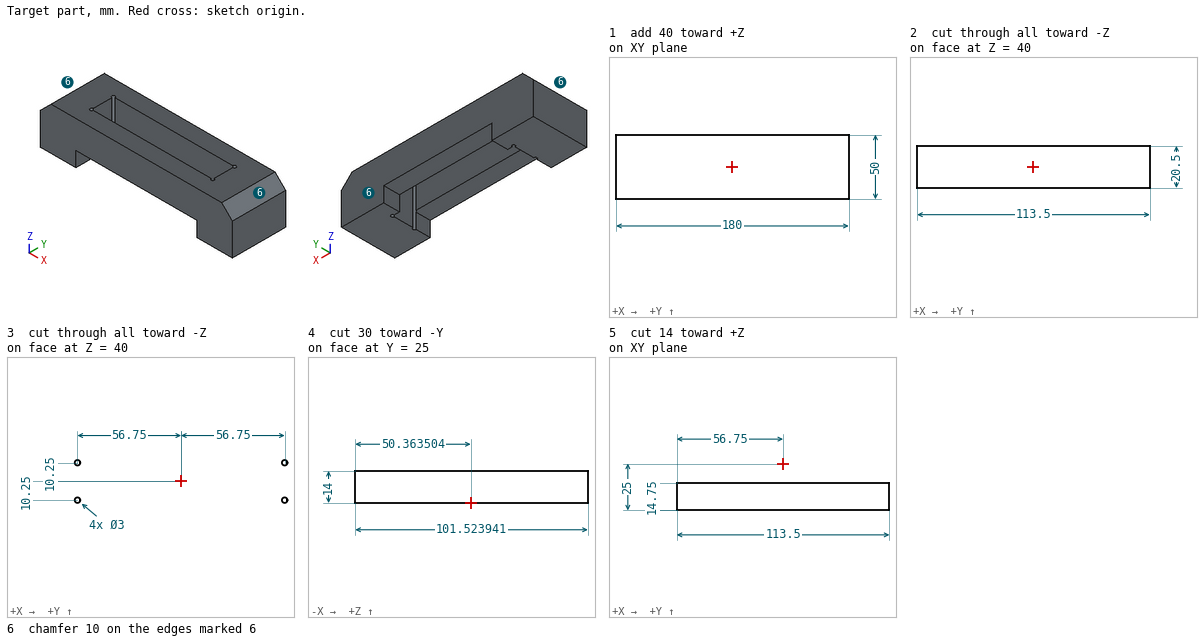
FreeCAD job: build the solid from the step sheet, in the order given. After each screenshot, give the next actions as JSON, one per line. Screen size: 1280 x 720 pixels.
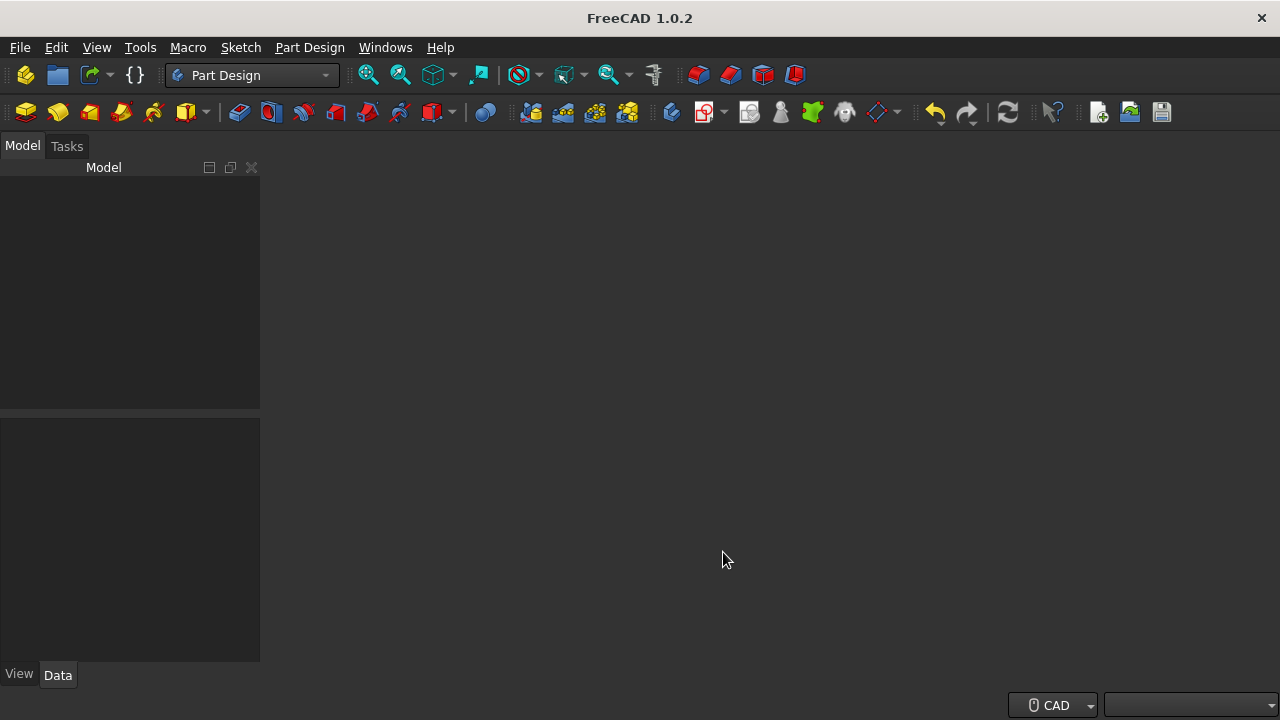
{"action": "left_click", "coordinate": [1098, 112]}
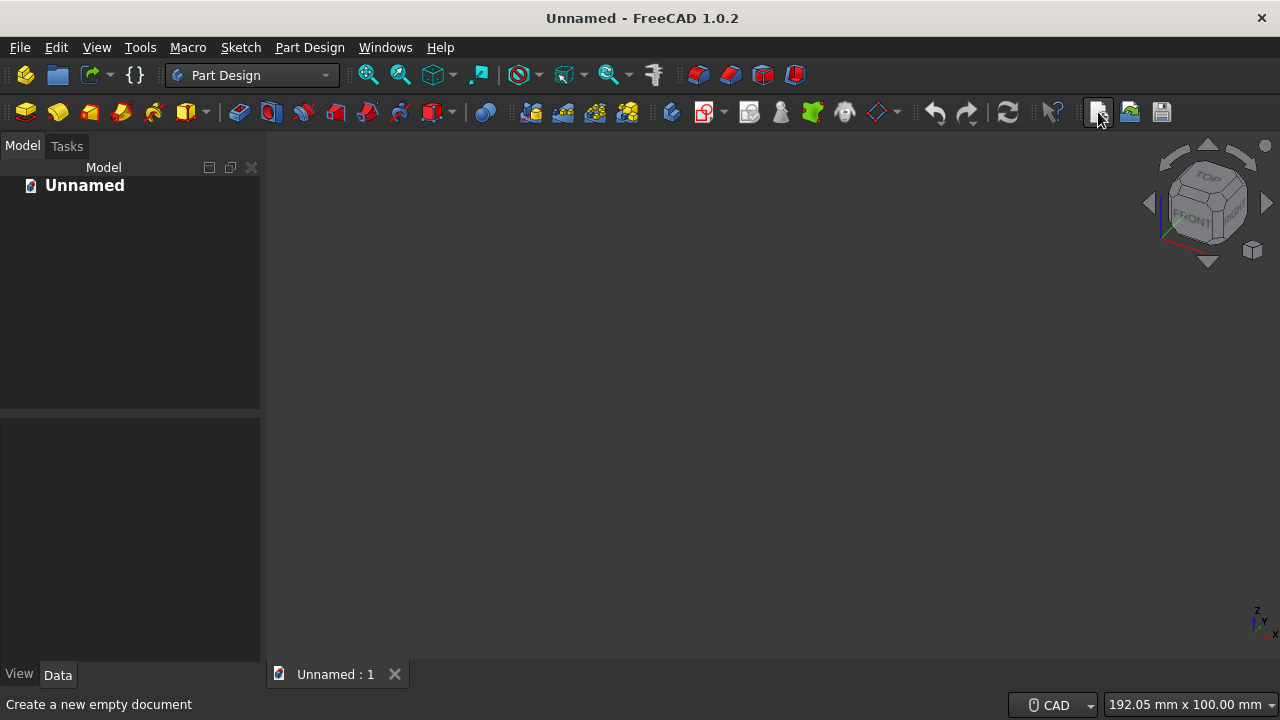
{"action": "left_click", "coordinate": [704, 112]}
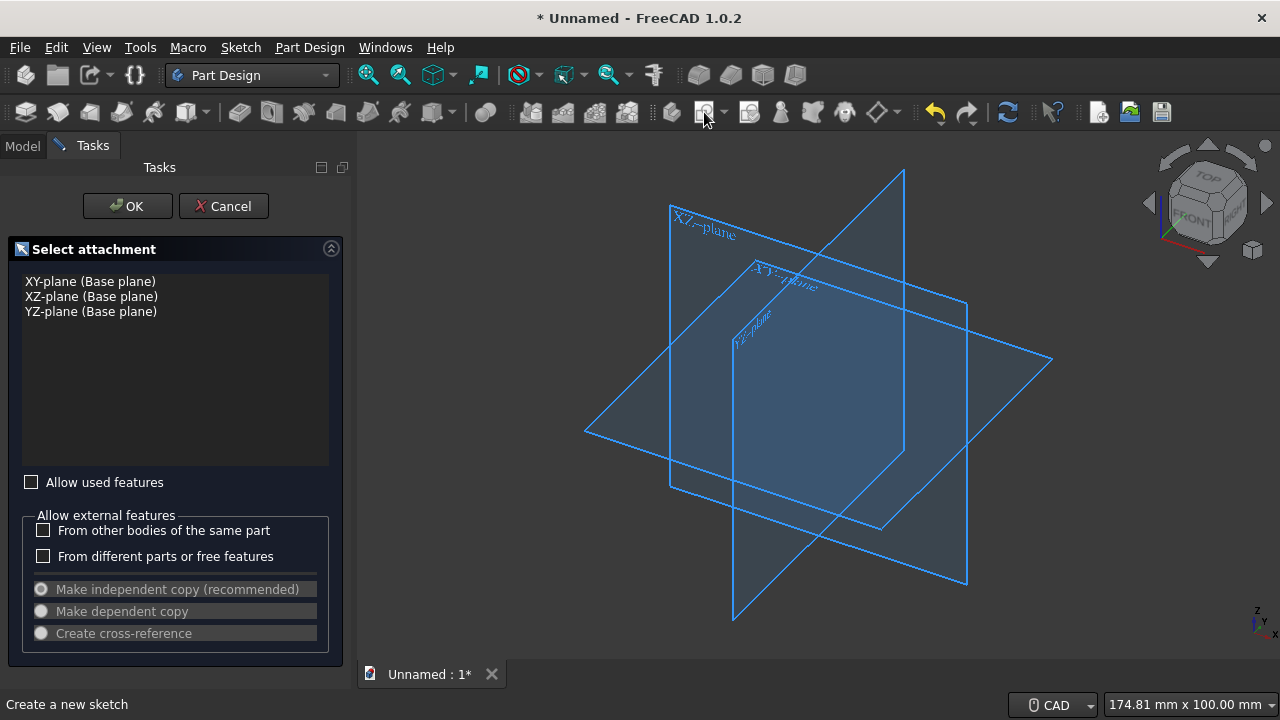
{"action": "left_click", "coordinate": [82, 282]}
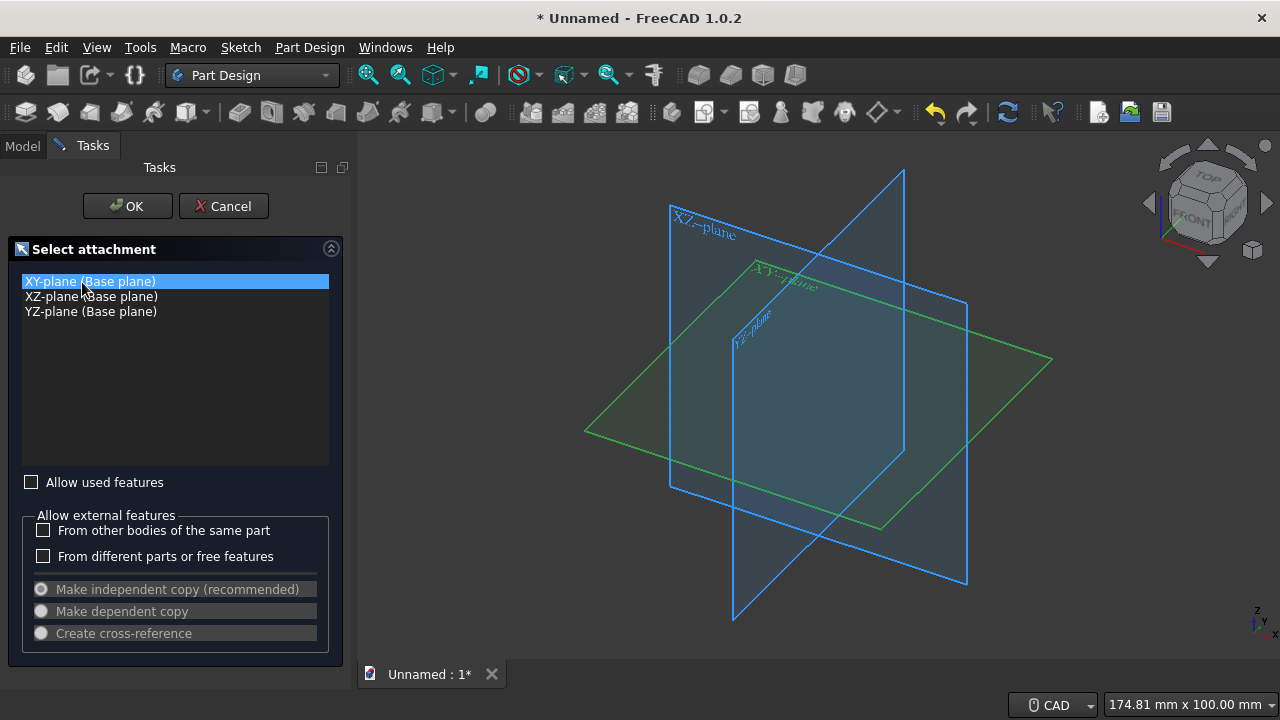
{"action": "left_click", "coordinate": [128, 206]}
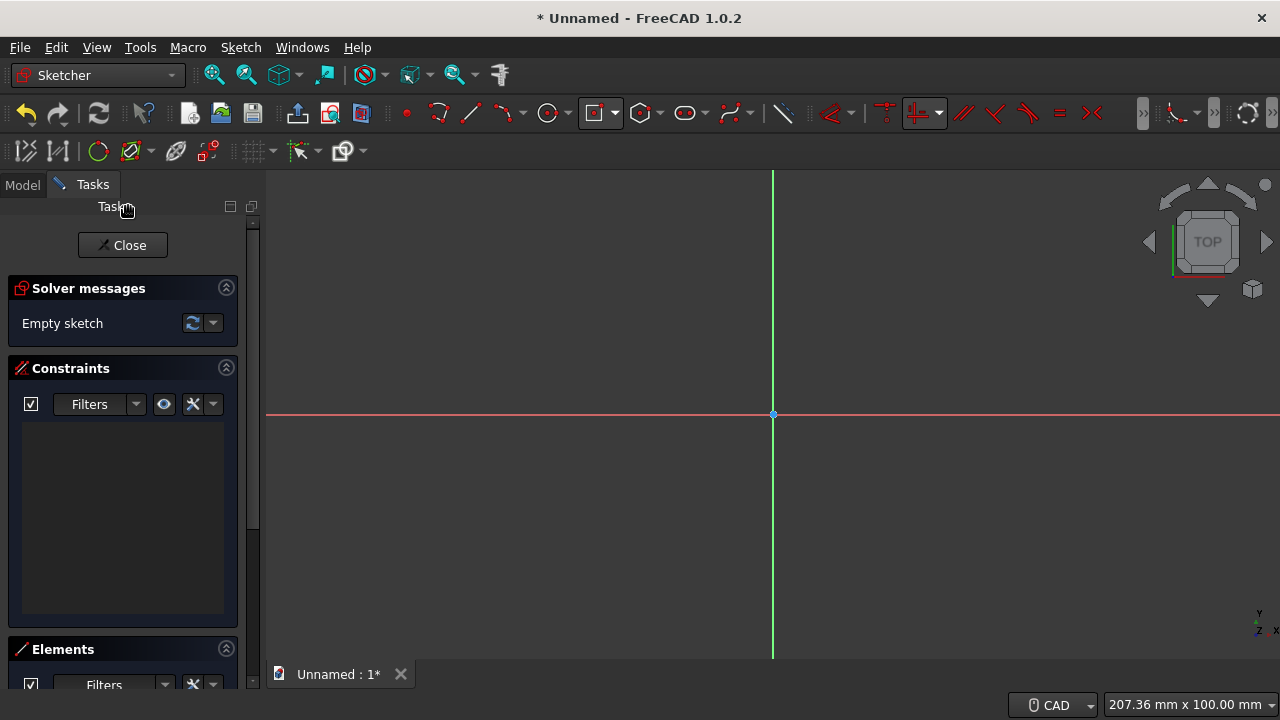
{"action": "scroll", "coordinate": [565, 414], "scroll_direction": "down", "scroll_amount": 2}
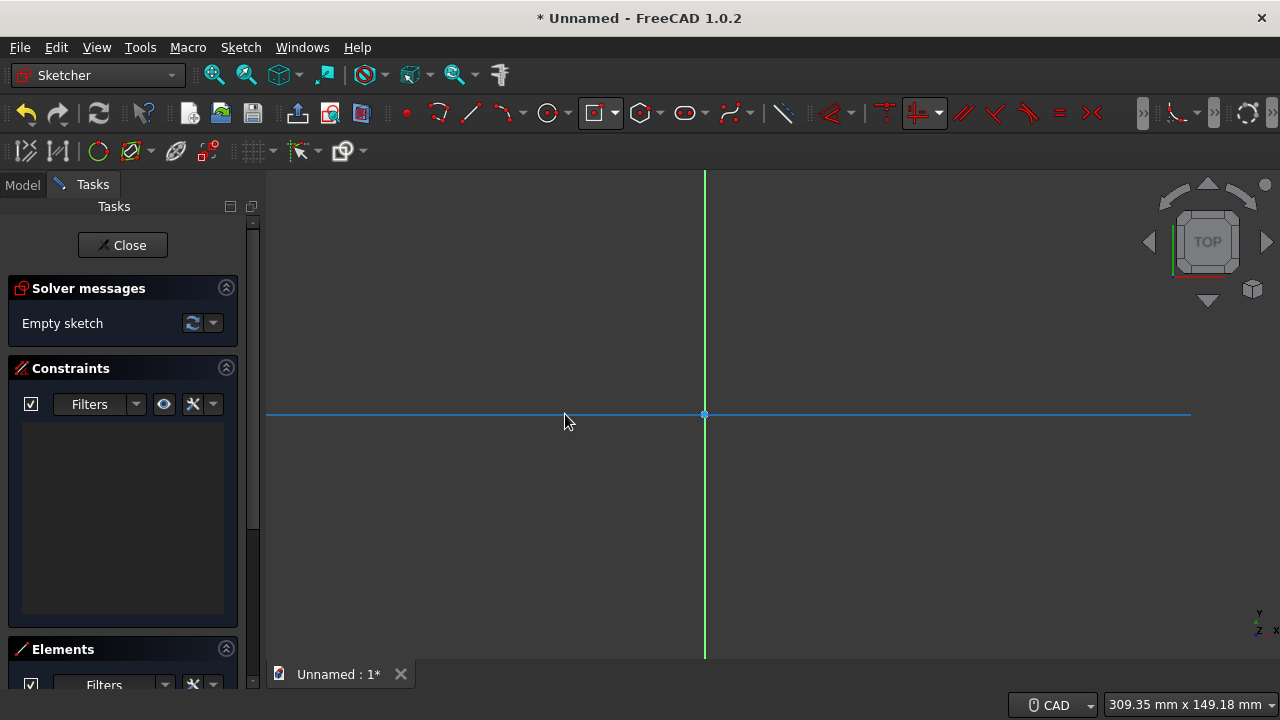
{"action": "left_click", "coordinate": [594, 114]}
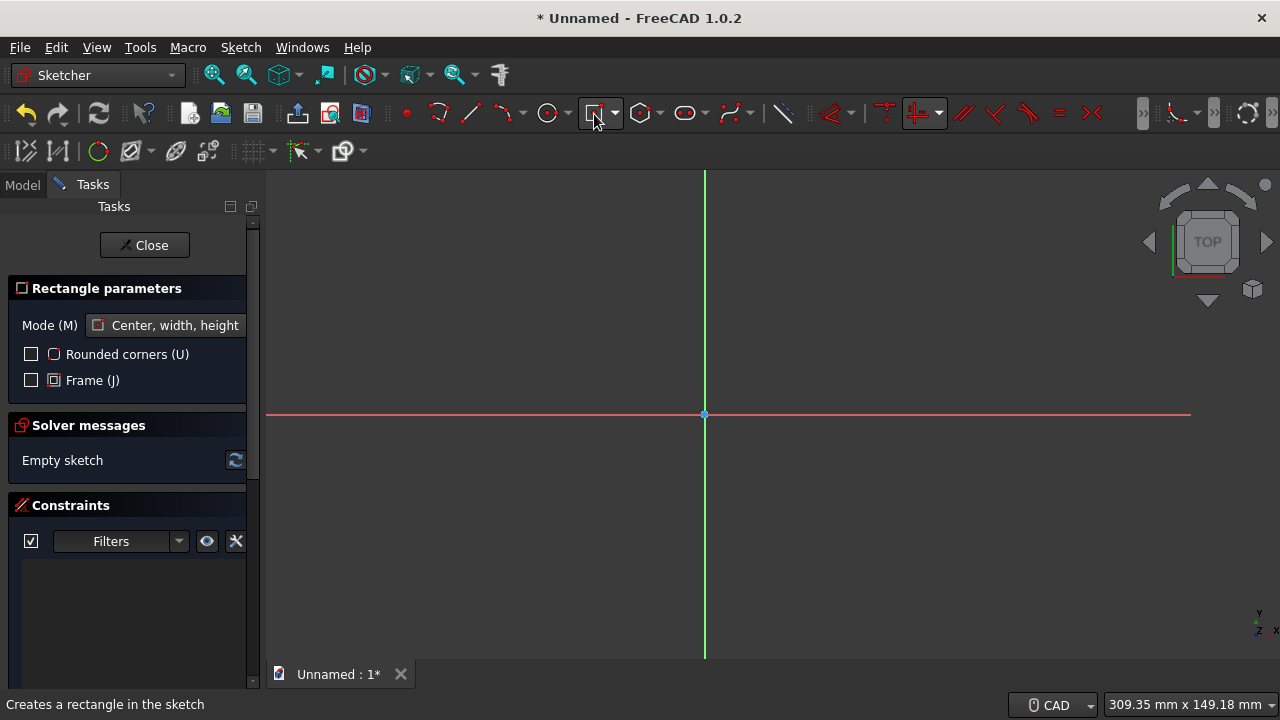
{"action": "left_click", "coordinate": [705, 414]}
{"action": "left_click", "coordinate": [1000, 333]}
{"action": "key", "text": "Escape"}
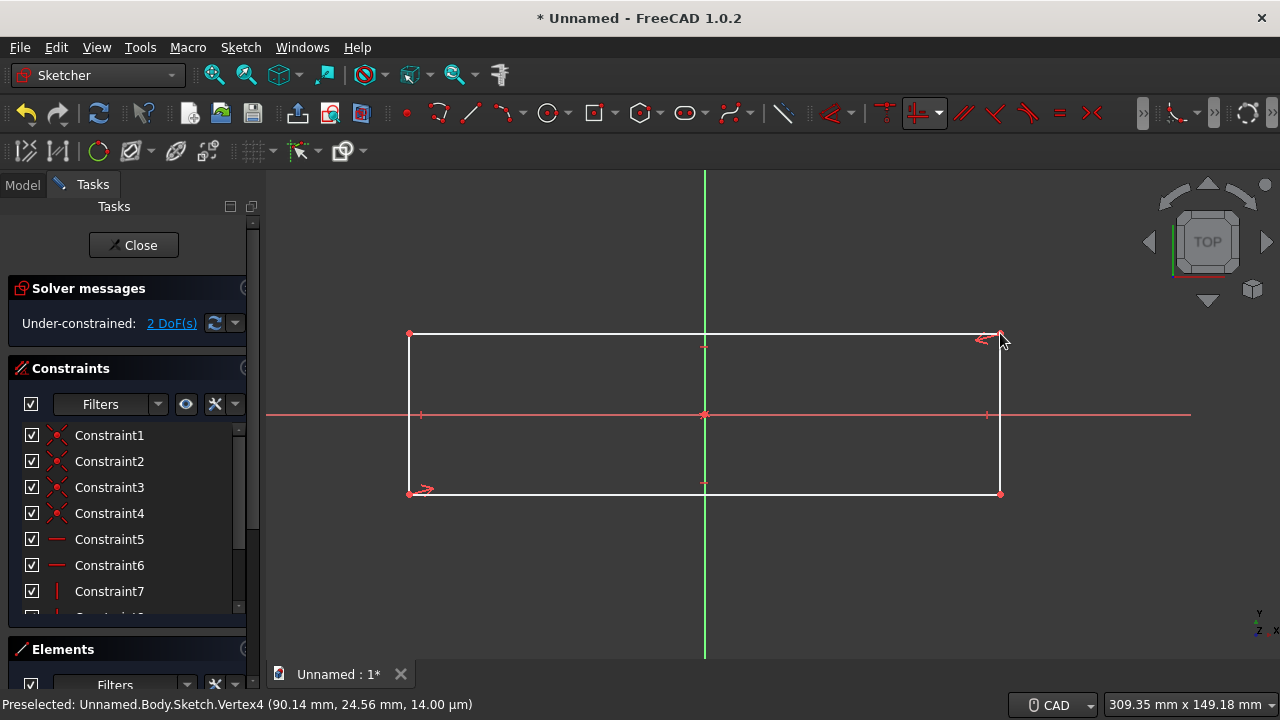
{"action": "left_click", "coordinate": [1000, 447]}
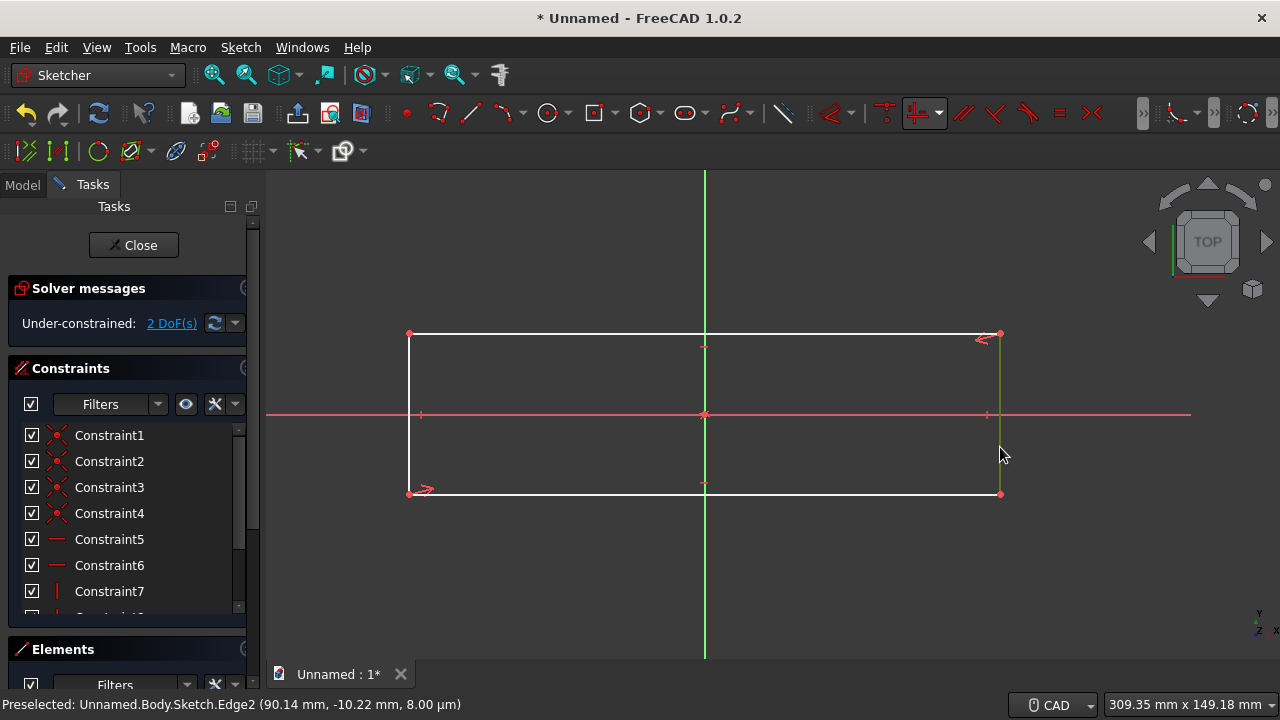
{"action": "left_click", "coordinate": [854, 114]}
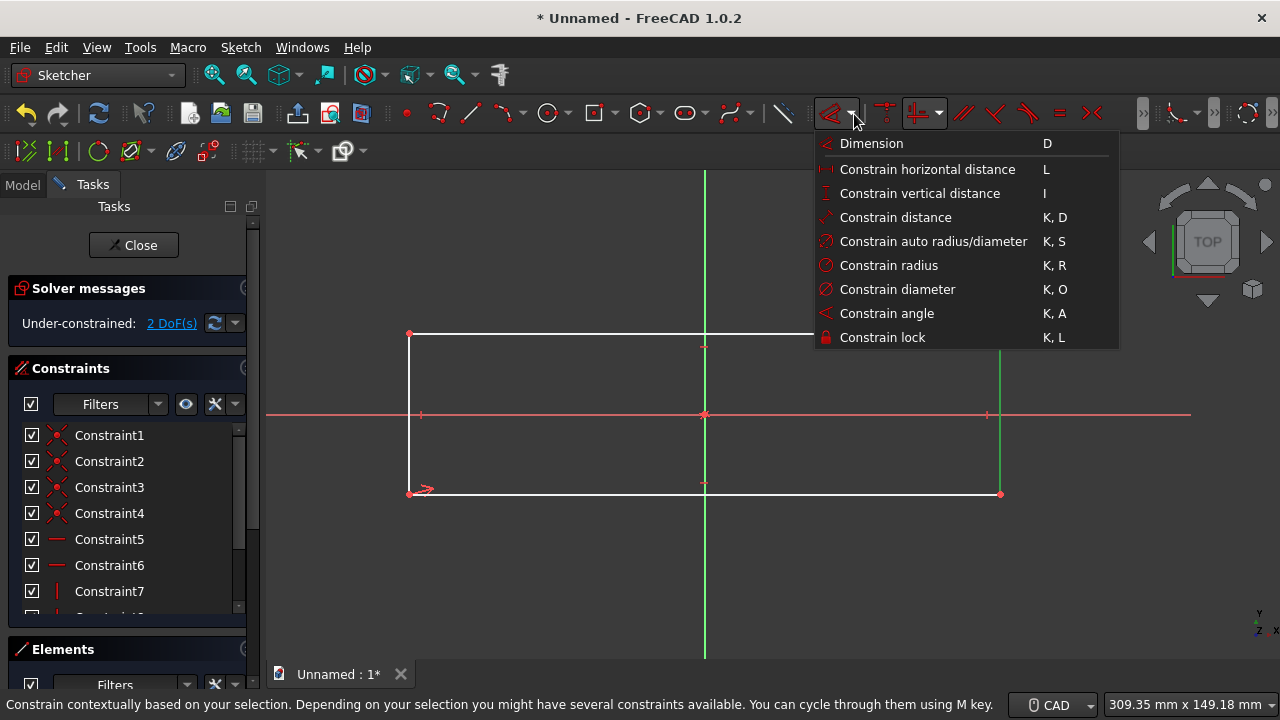
{"action": "left_click", "coordinate": [967, 193]}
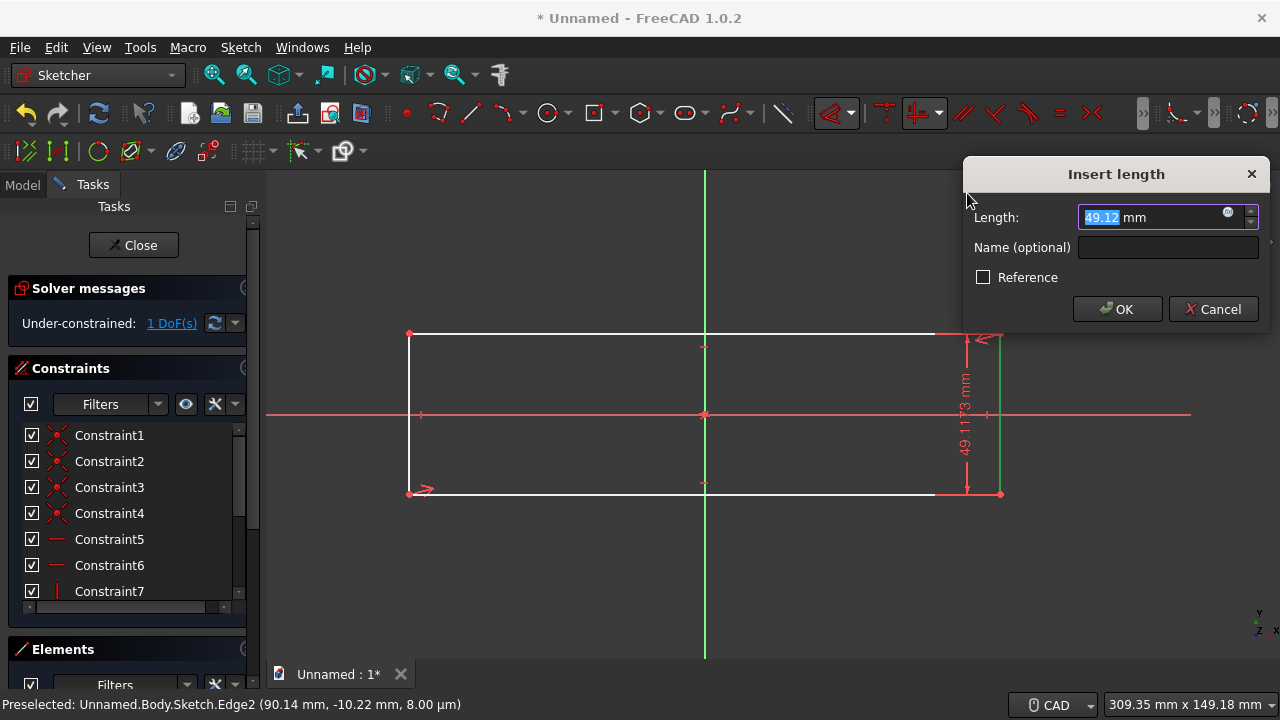
{"action": "type", "text": "50"}
{"action": "key", "text": "Return"}